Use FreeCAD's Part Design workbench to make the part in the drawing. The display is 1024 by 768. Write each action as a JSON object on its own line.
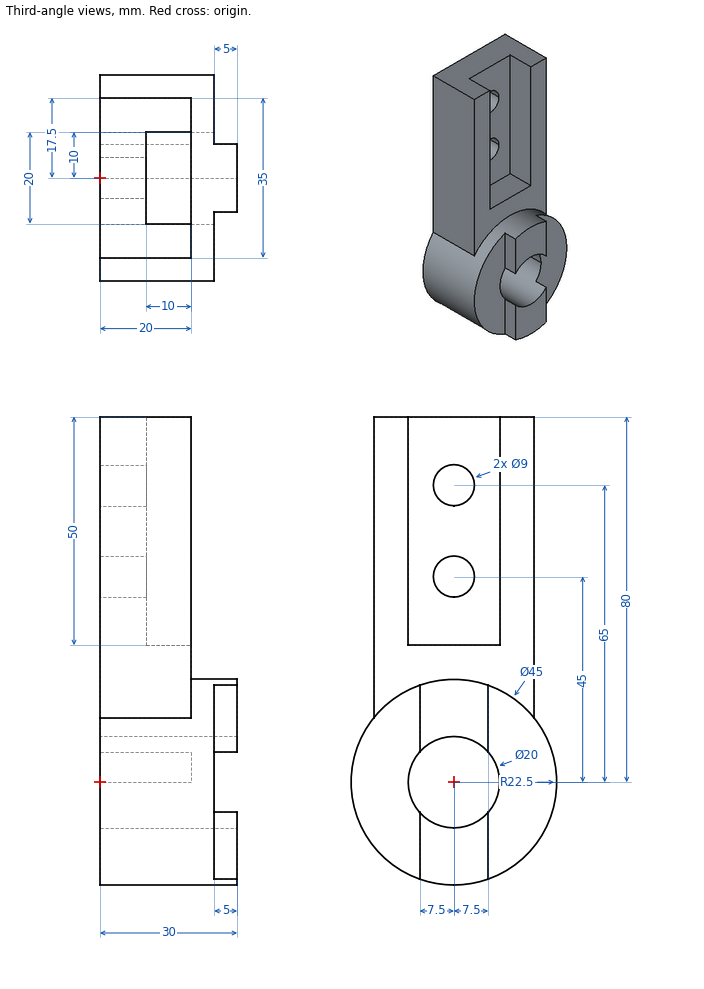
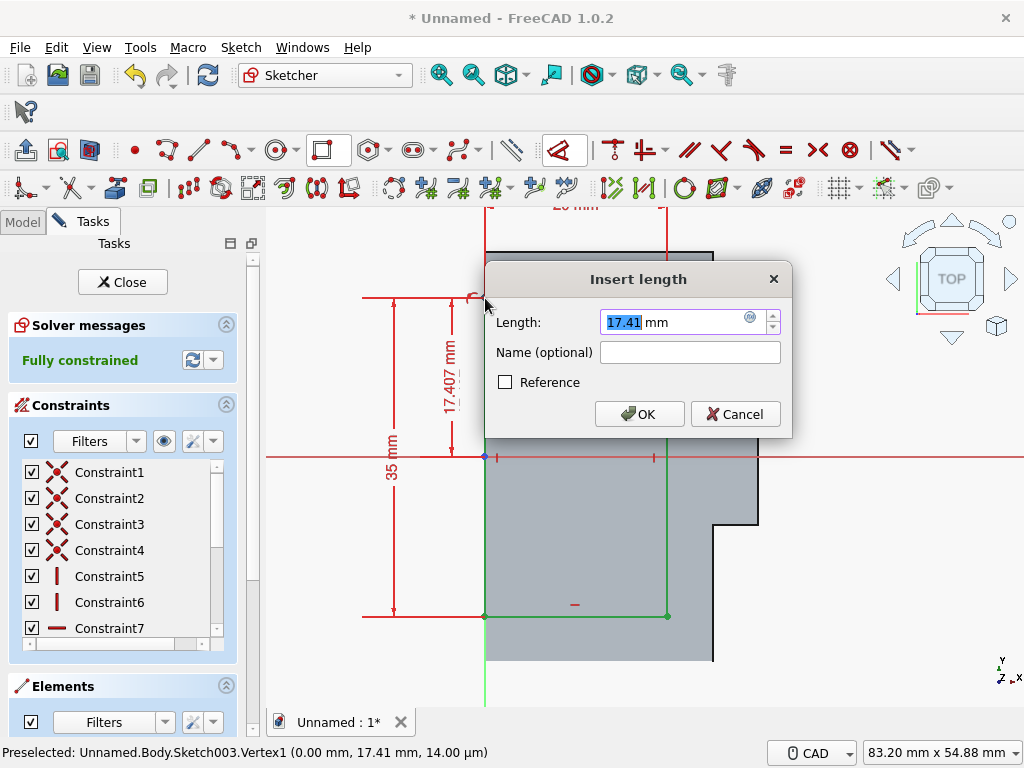
{"action": "type", "text": "17.5"}
{"action": "key", "text": "Return"}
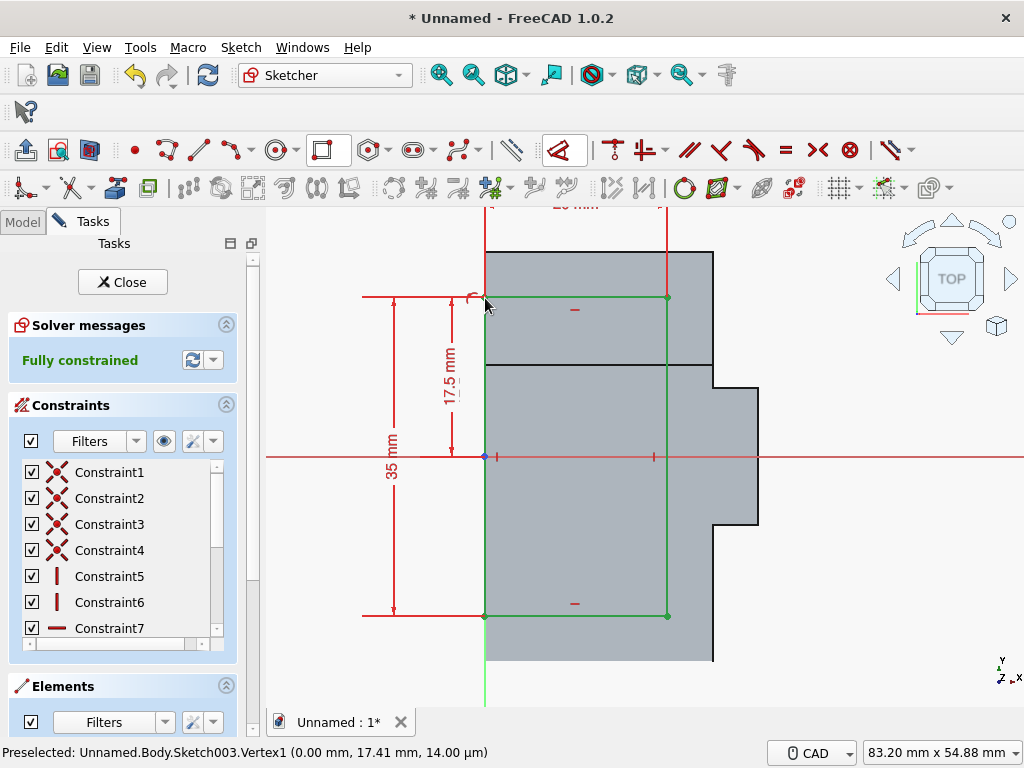
{"action": "left_click", "coordinate": [123, 282]}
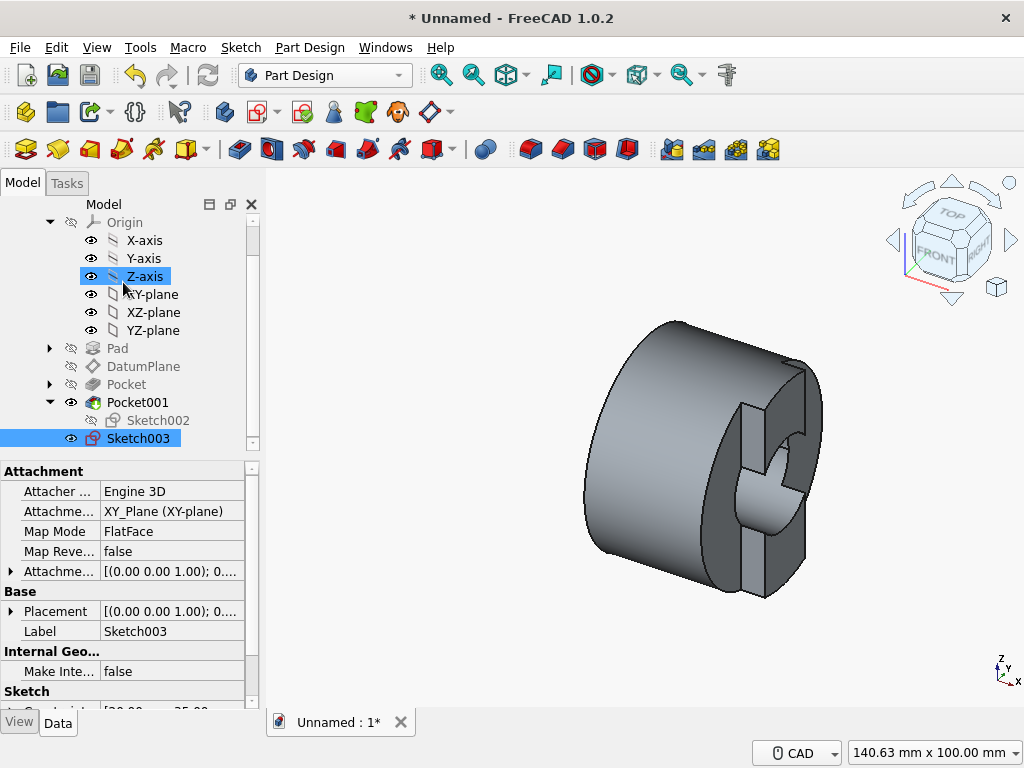
{"action": "left_click", "coordinate": [26, 150]}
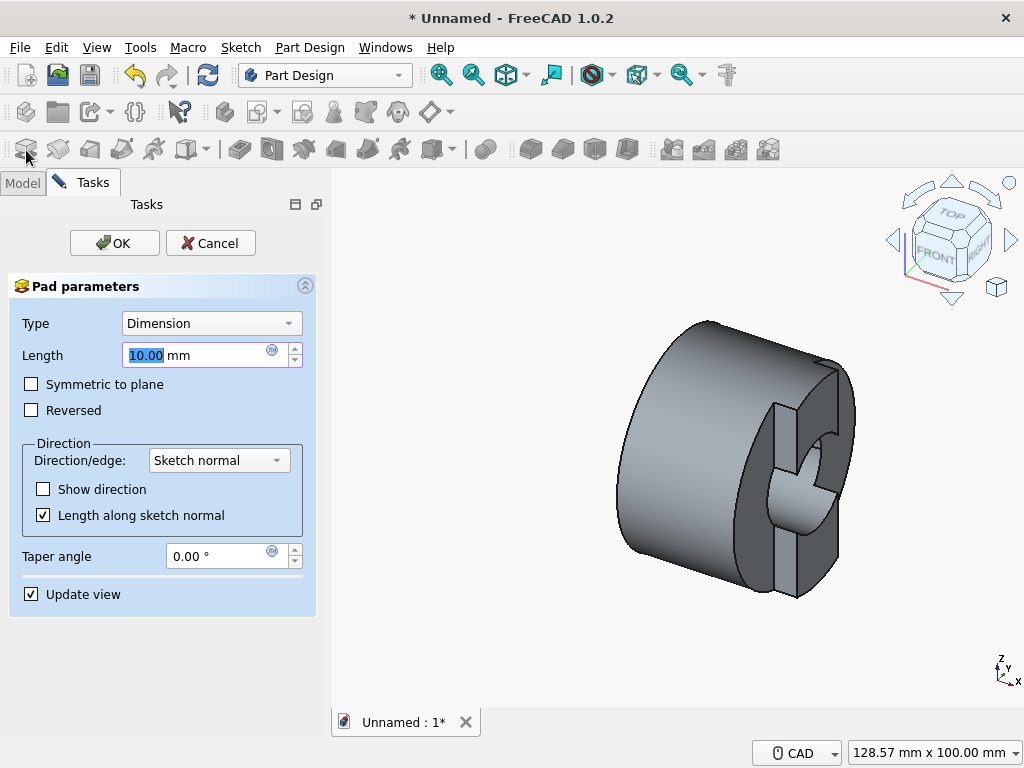
{"action": "type", "text": "80"}
{"action": "key", "text": "Tab"}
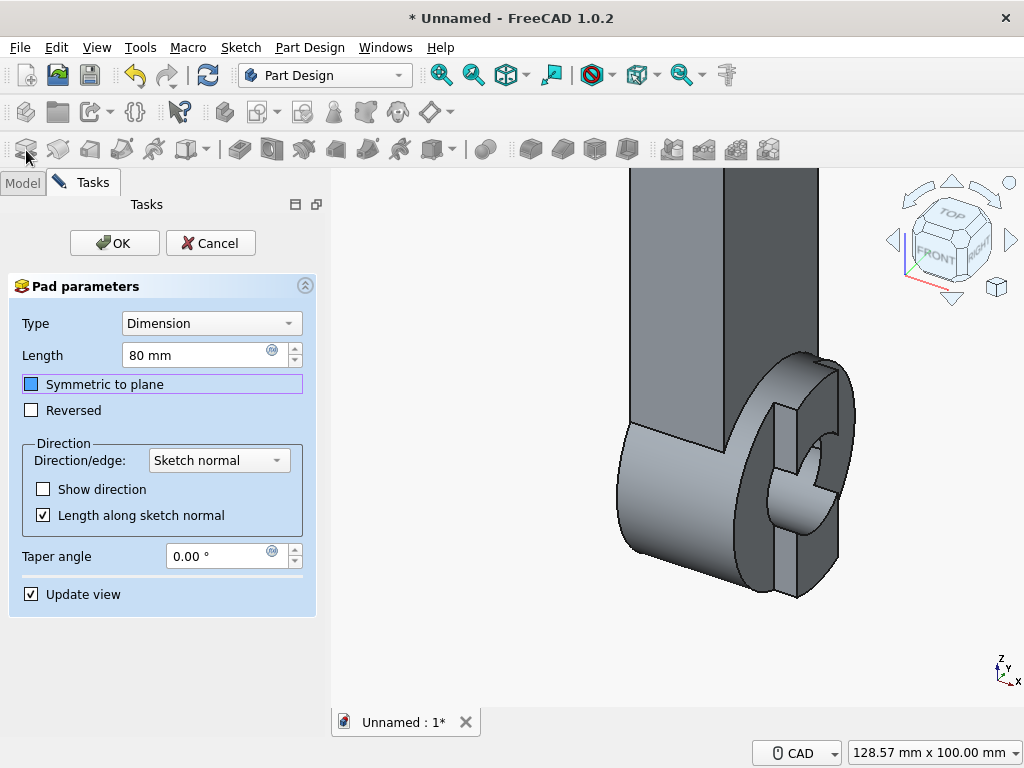
{"action": "left_click", "coordinate": [115, 243]}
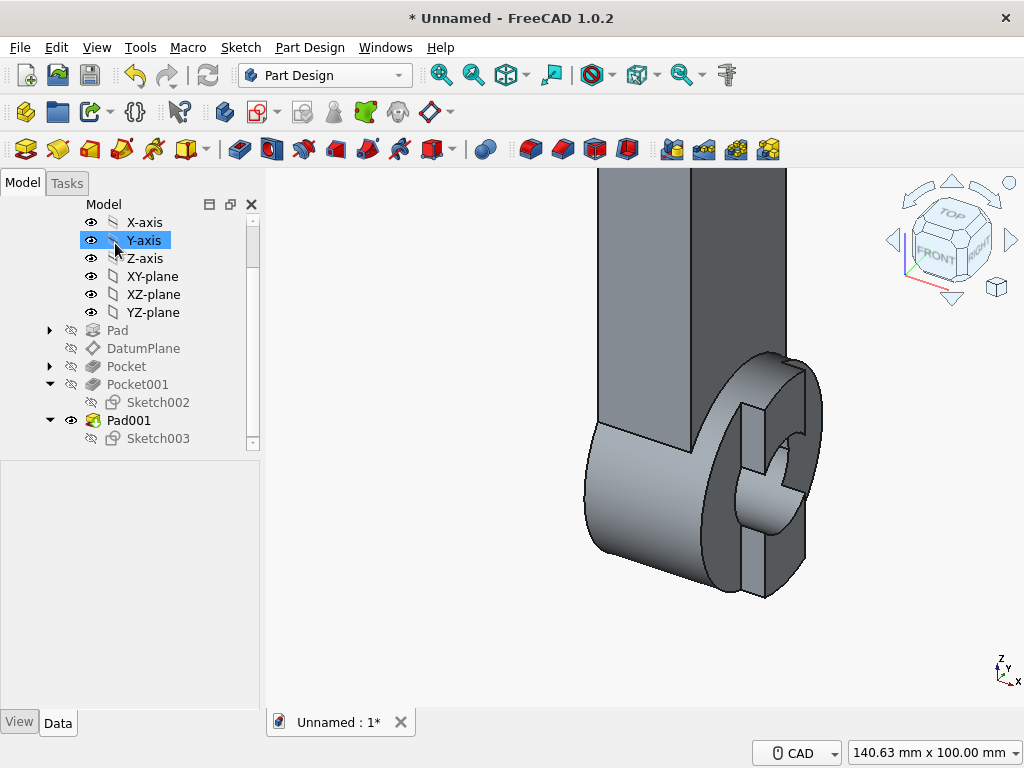
{"action": "left_click", "coordinate": [442, 76]}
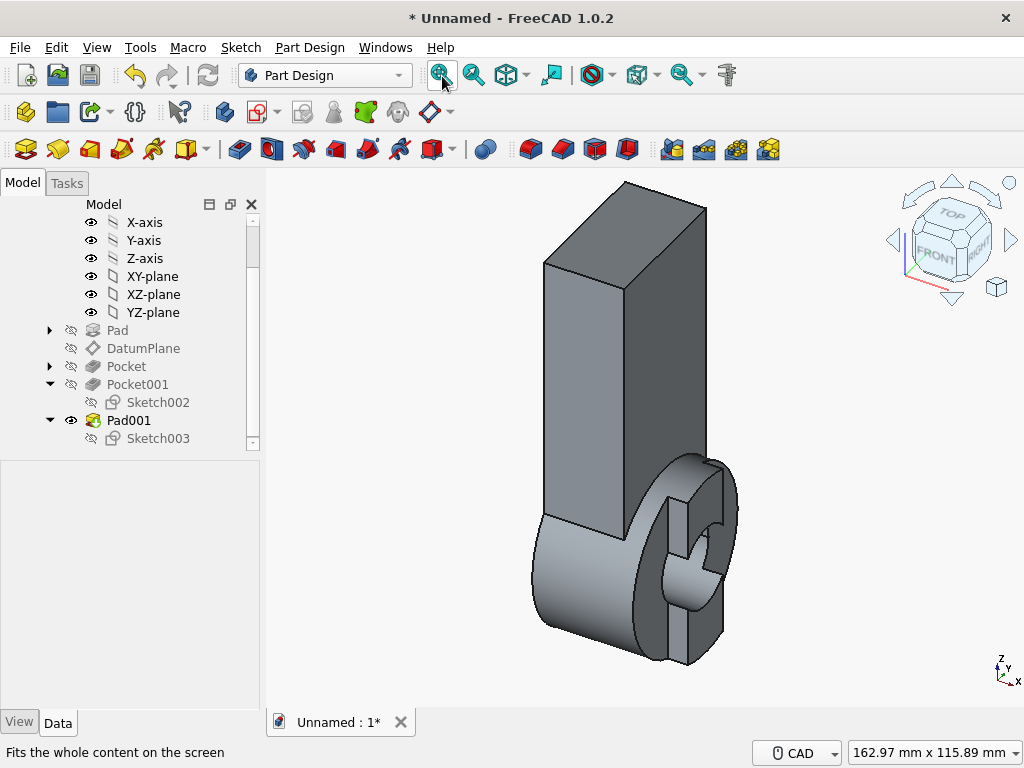
{"action": "scroll", "coordinate": [160, 326], "scroll_direction": "down", "scroll_amount": 3}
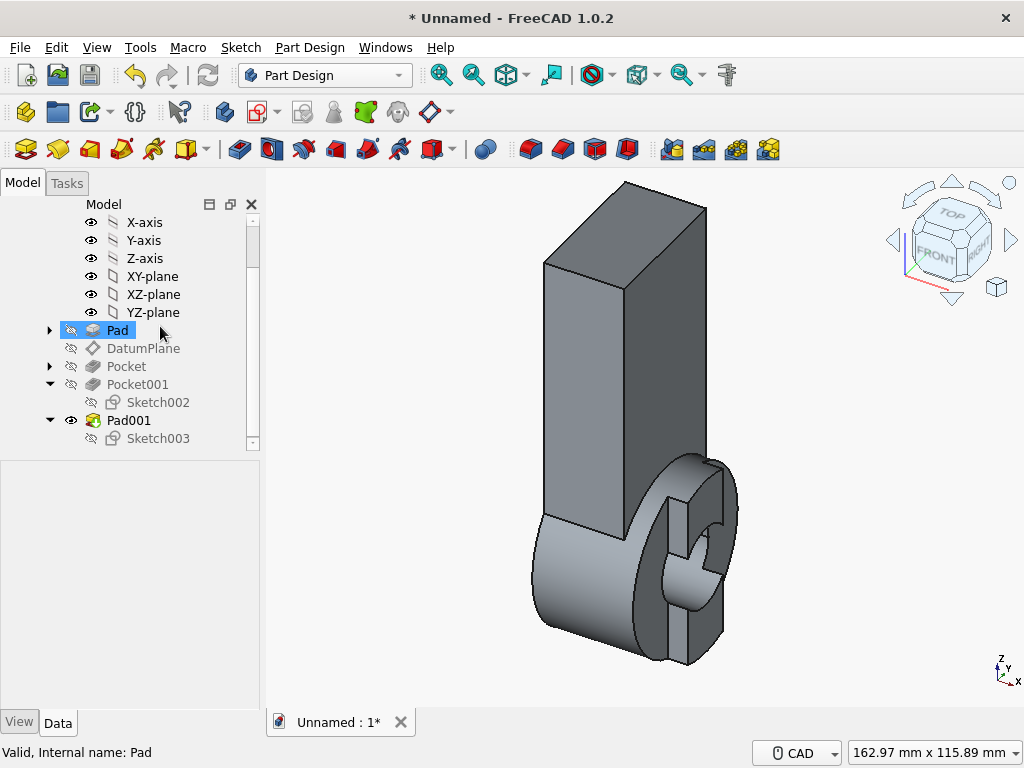
{"action": "scroll", "coordinate": [160, 326], "scroll_direction": "up", "scroll_amount": 15}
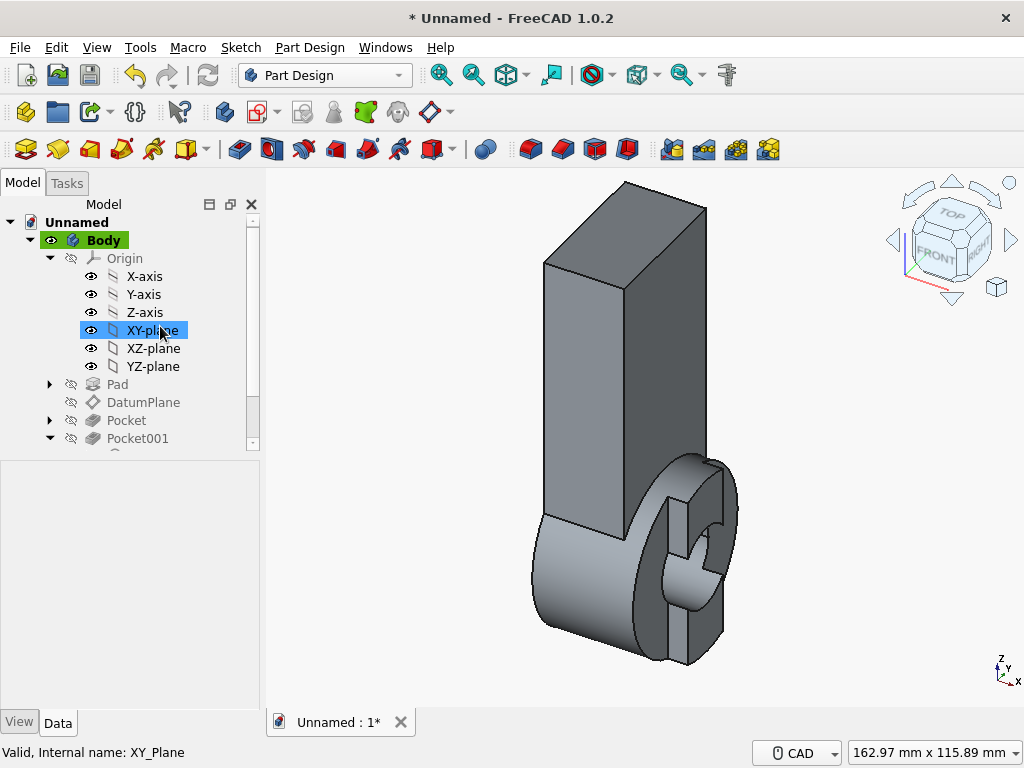
{"action": "left_click", "coordinate": [136, 366]}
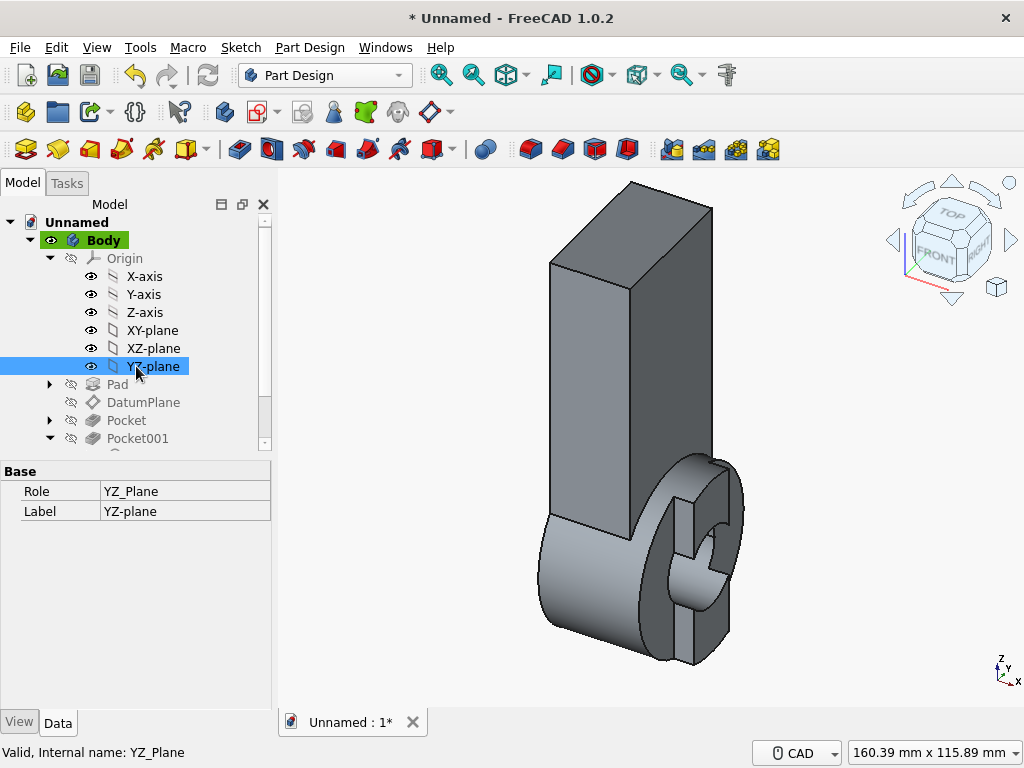
{"action": "left_click", "coordinate": [430, 112]}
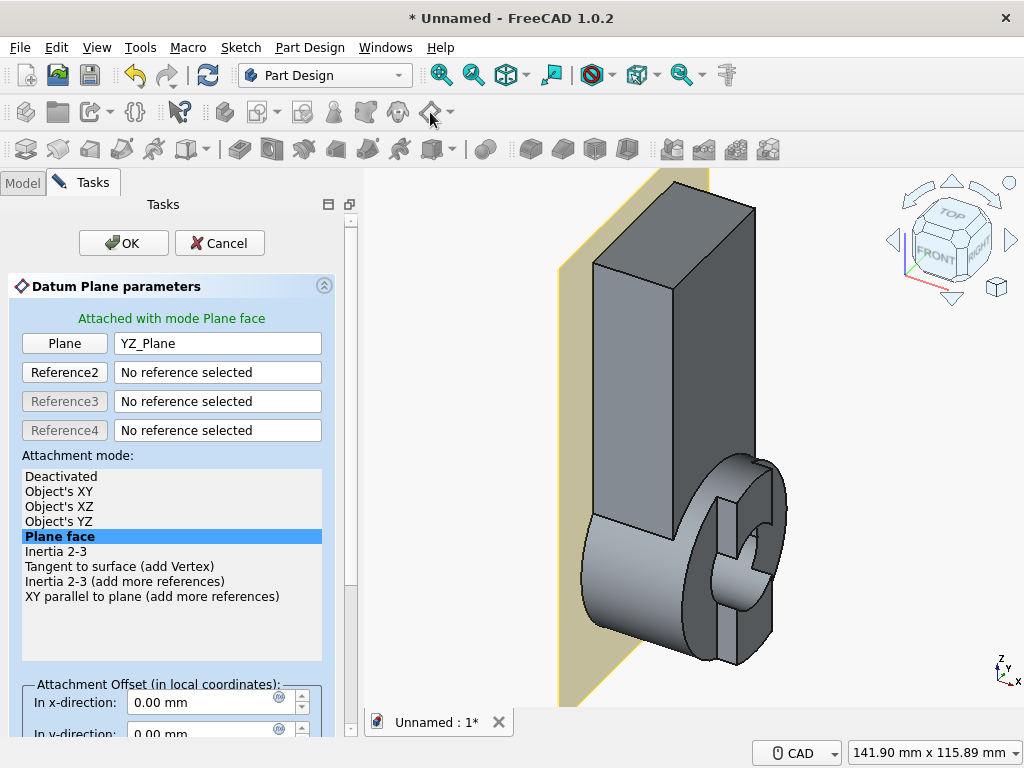
{"action": "scroll", "coordinate": [351, 475], "scroll_direction": "down", "scroll_amount": 2}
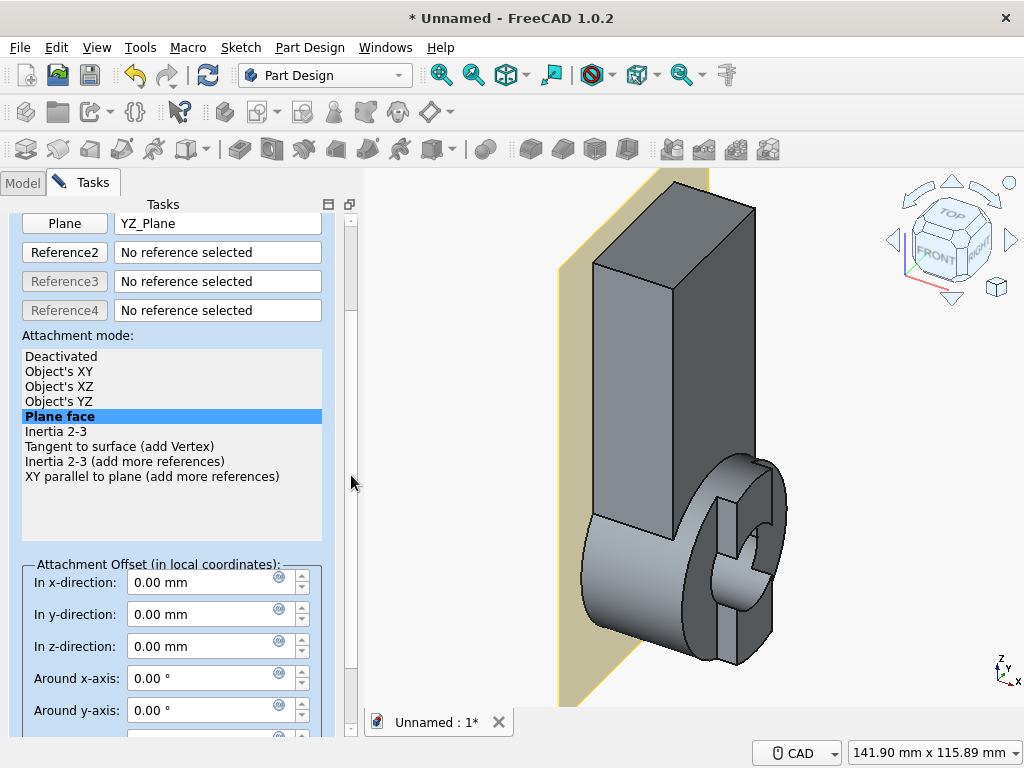
{"action": "triple_click", "coordinate": [210, 646]}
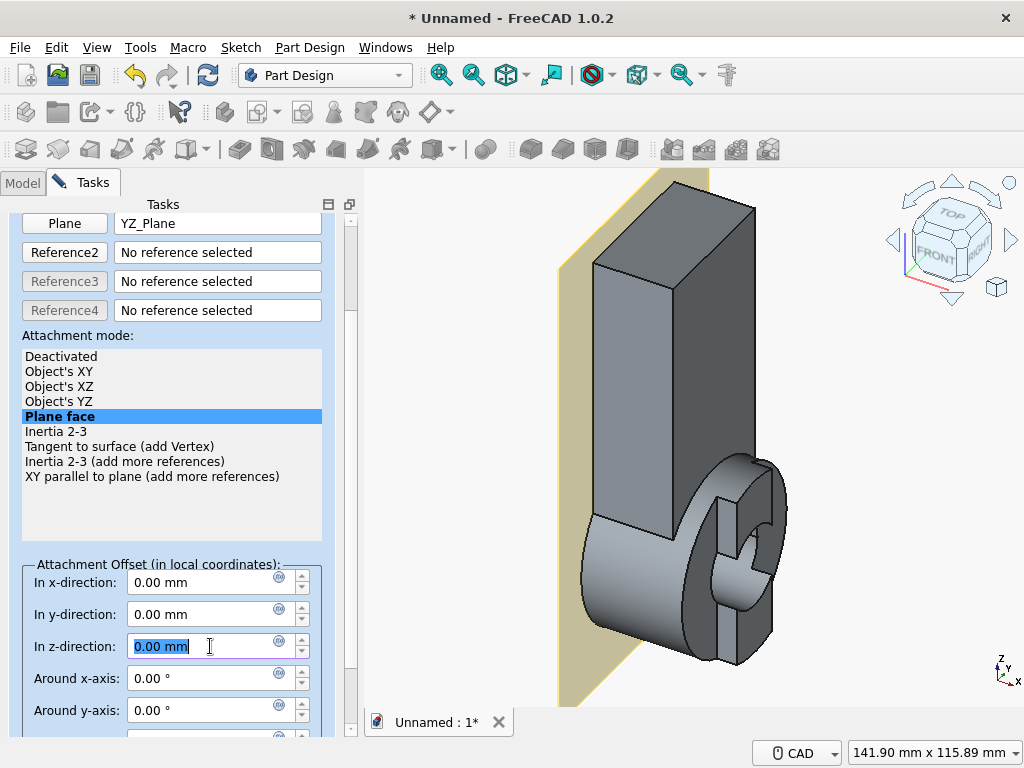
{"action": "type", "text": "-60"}
{"action": "key", "text": "Tab"}